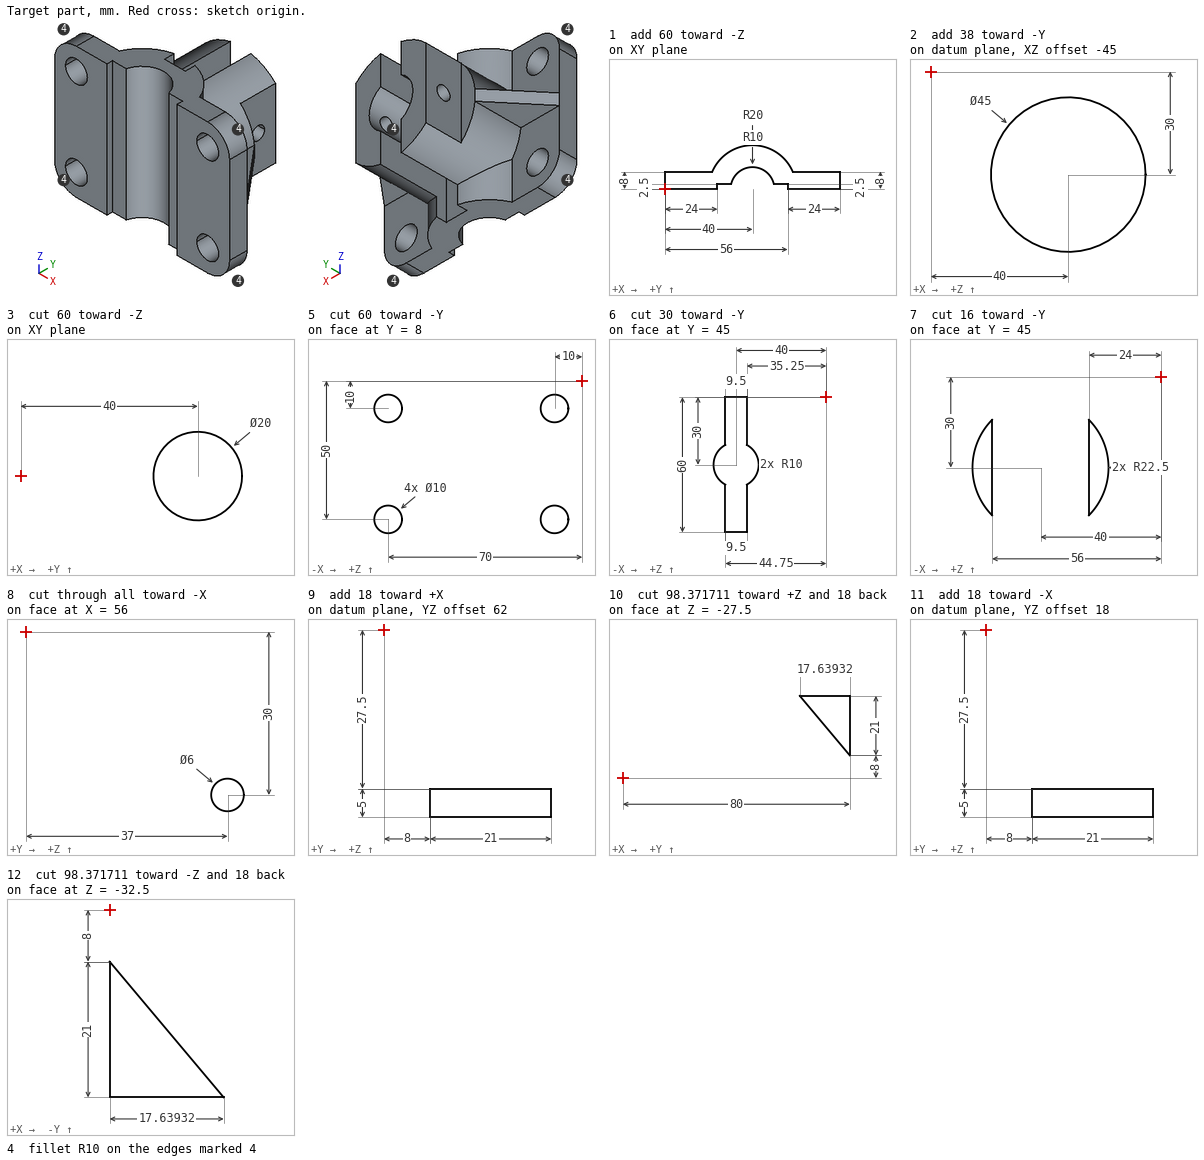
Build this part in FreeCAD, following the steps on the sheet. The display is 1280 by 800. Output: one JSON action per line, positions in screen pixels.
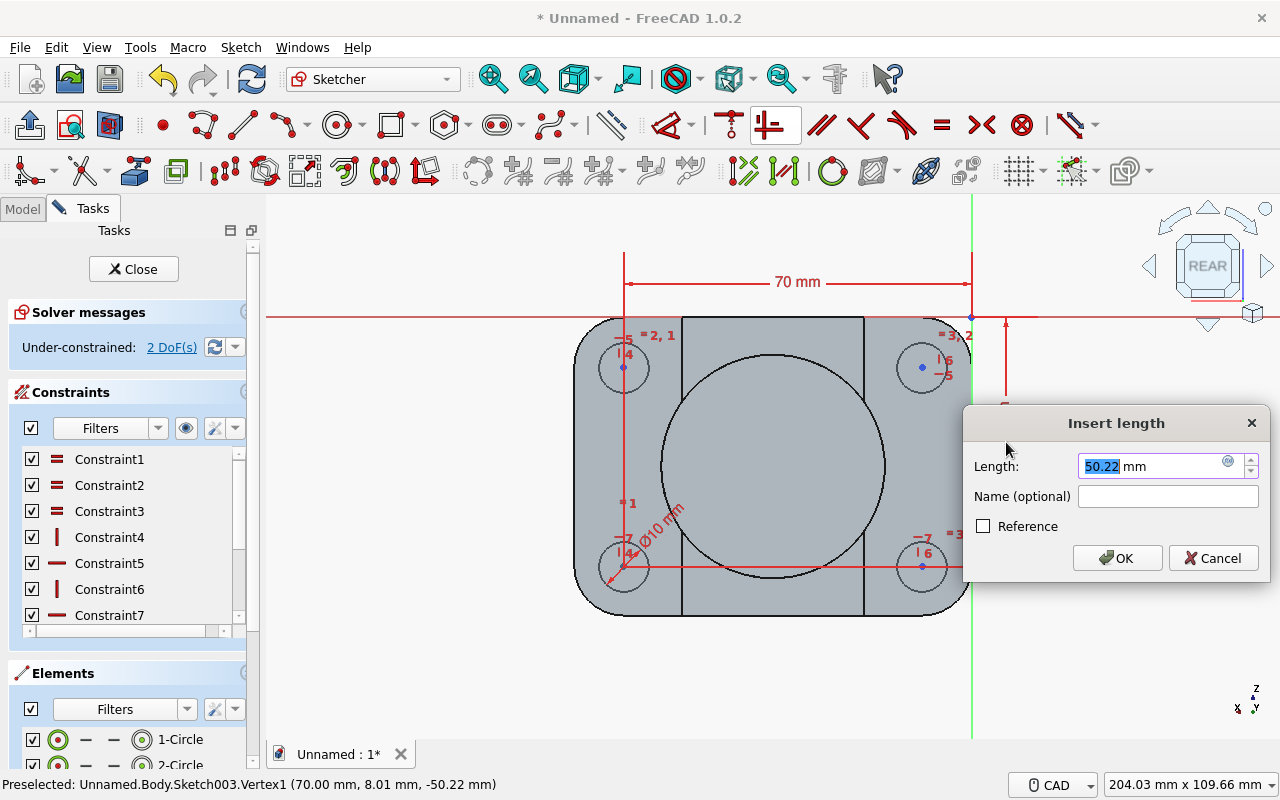
{"action": "type", "text": "50"}
{"action": "key", "text": "Return"}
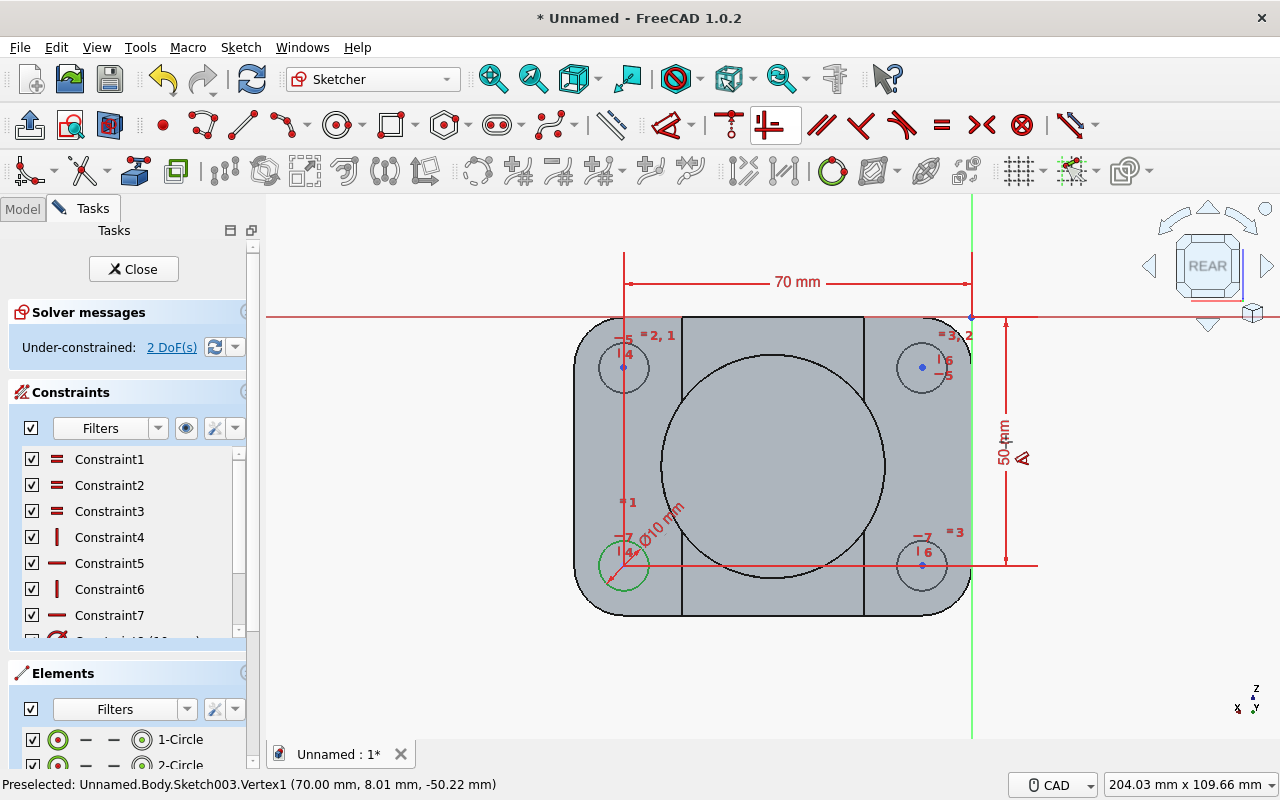
{"action": "left_click", "coordinate": [624, 368]}
{"action": "left_click", "coordinate": [1006, 343]}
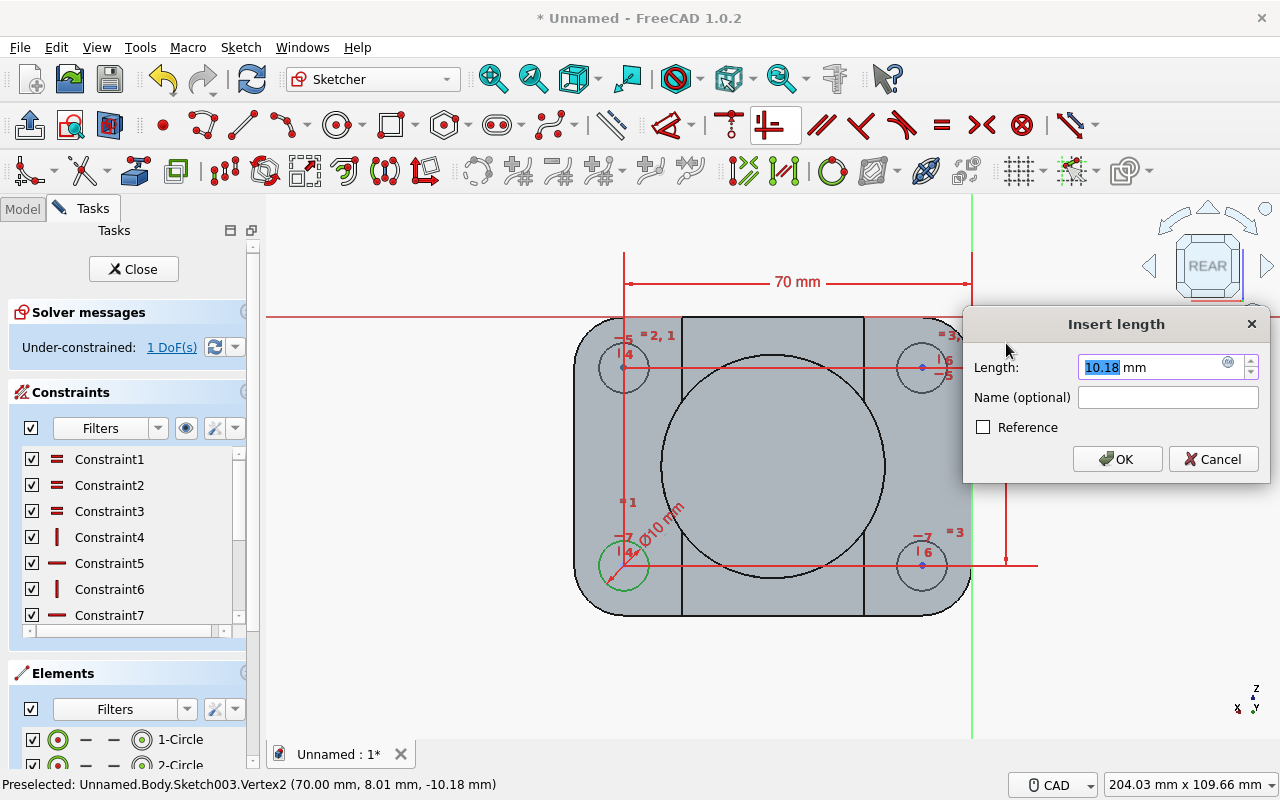
{"action": "type", "text": "10"}
{"action": "key", "text": "Return"}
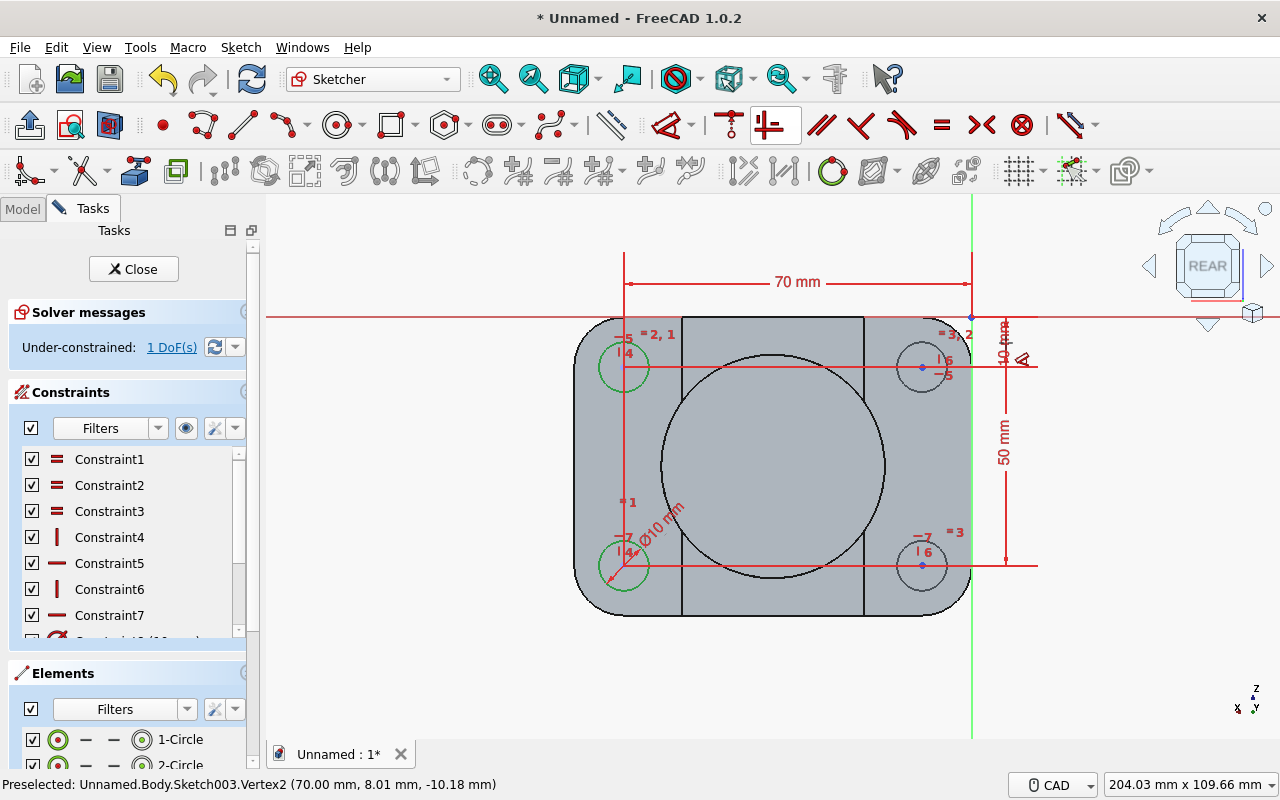
{"action": "left_click", "coordinate": [922, 367]}
{"action": "left_click", "coordinate": [947, 283]}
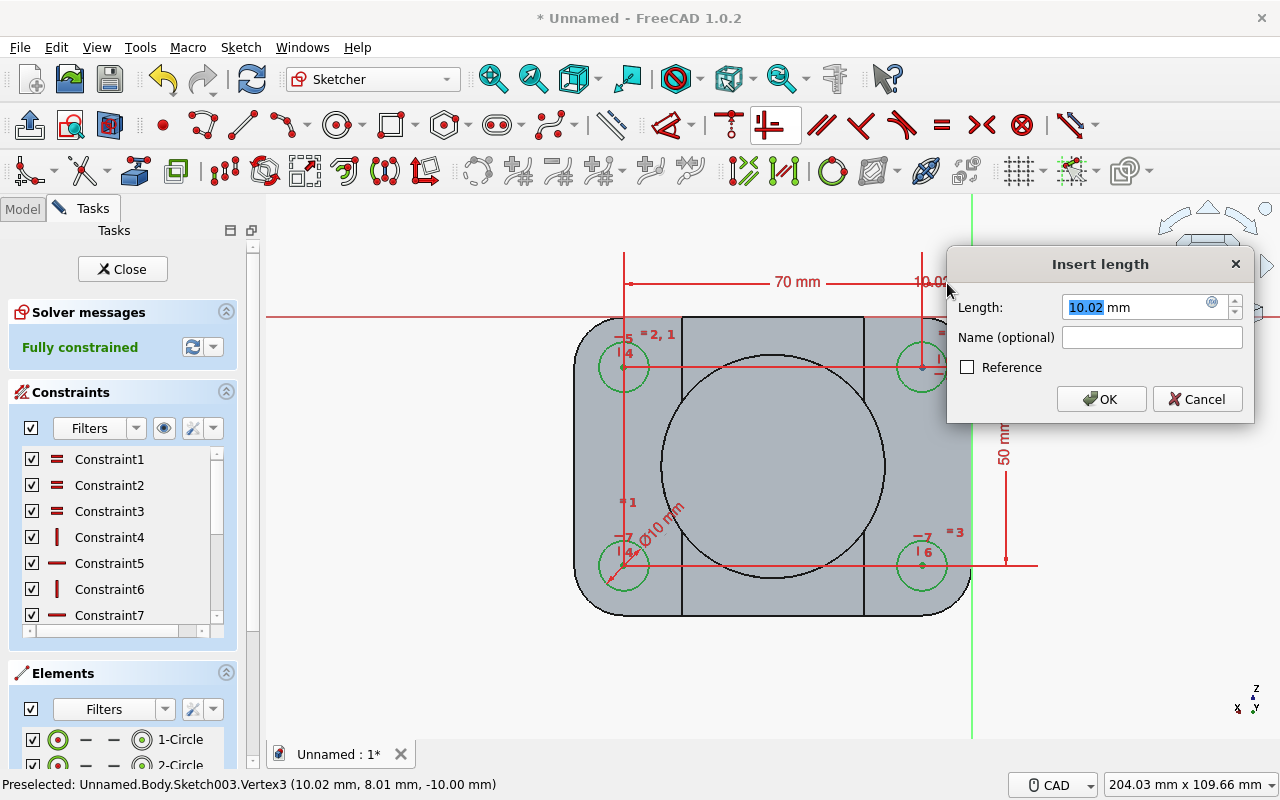
{"action": "type", "text": "10"}
{"action": "key", "text": "Return"}
{"action": "key", "text": "Escape"}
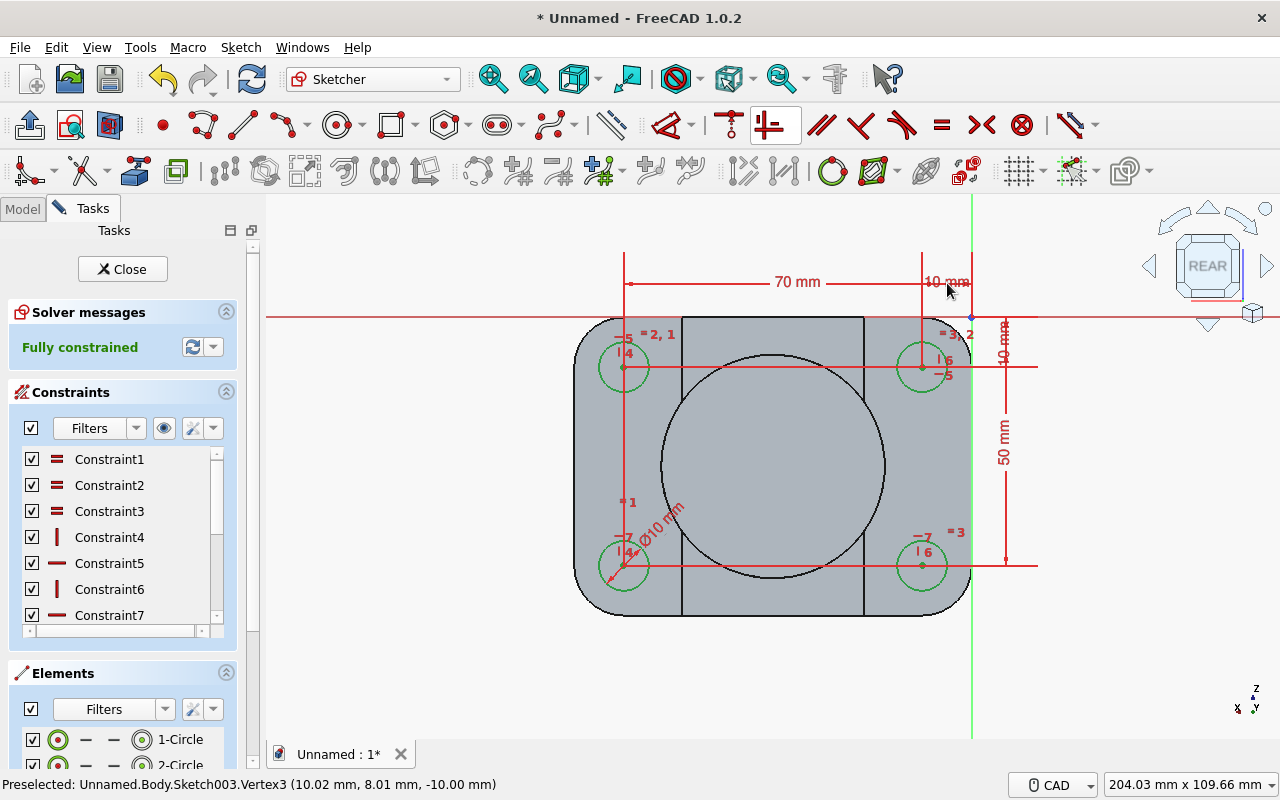
{"action": "left_click", "coordinate": [123, 269]}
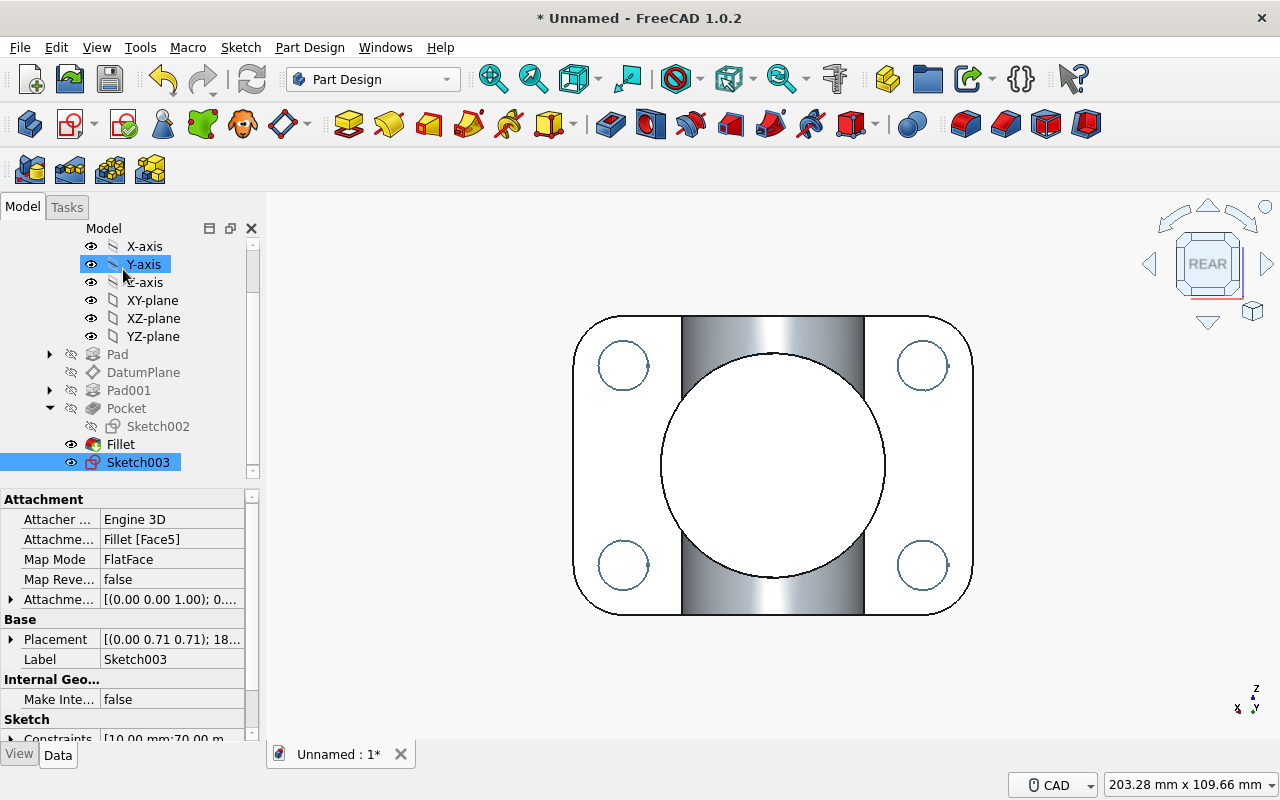
{"action": "left_click", "coordinate": [612, 124]}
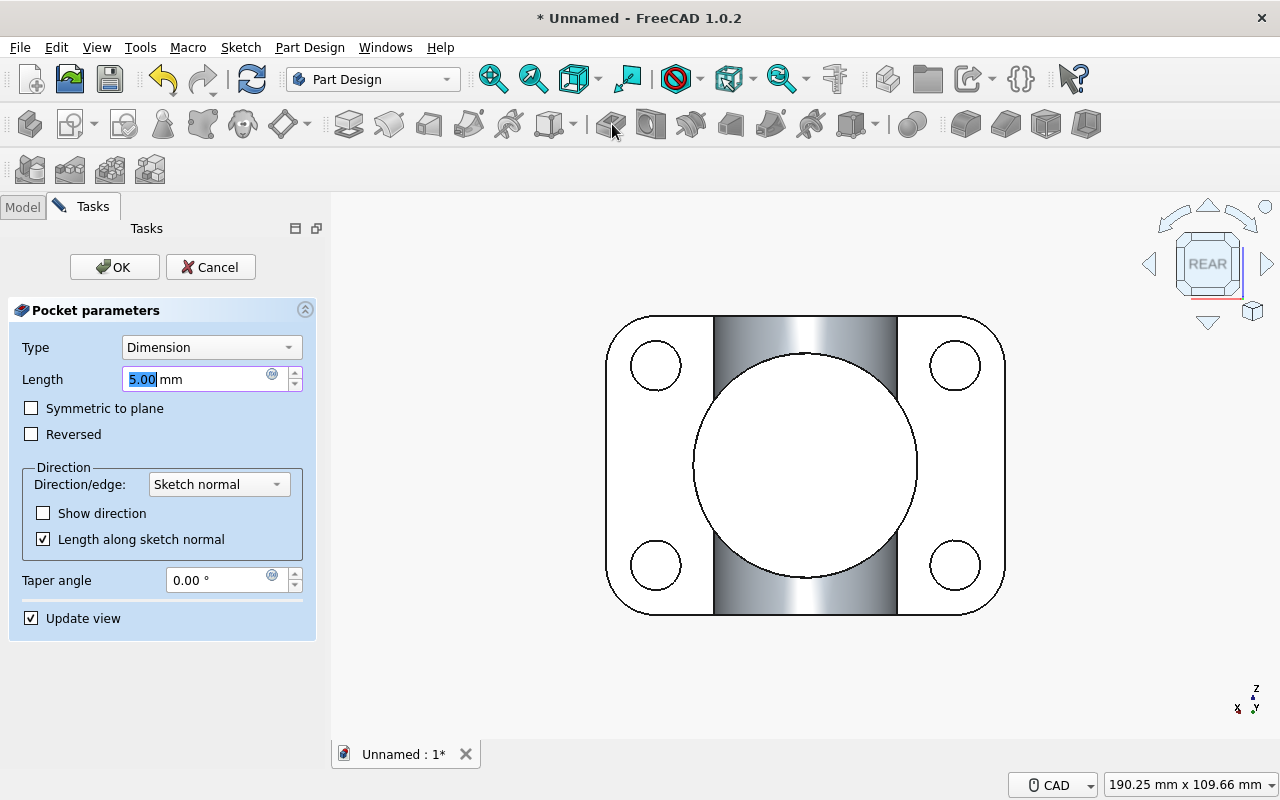
{"action": "type", "text": "60"}
{"action": "key", "text": "Tab"}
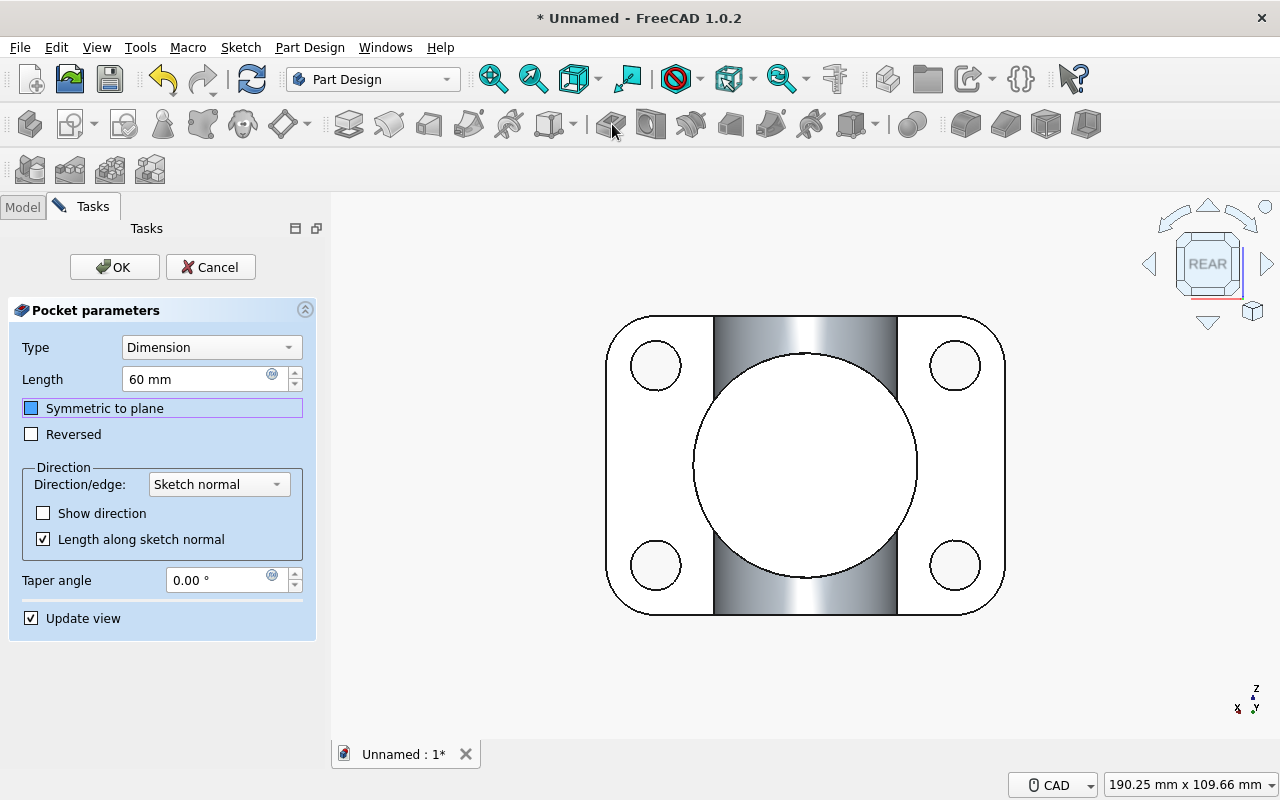
{"action": "left_click", "coordinate": [115, 267]}